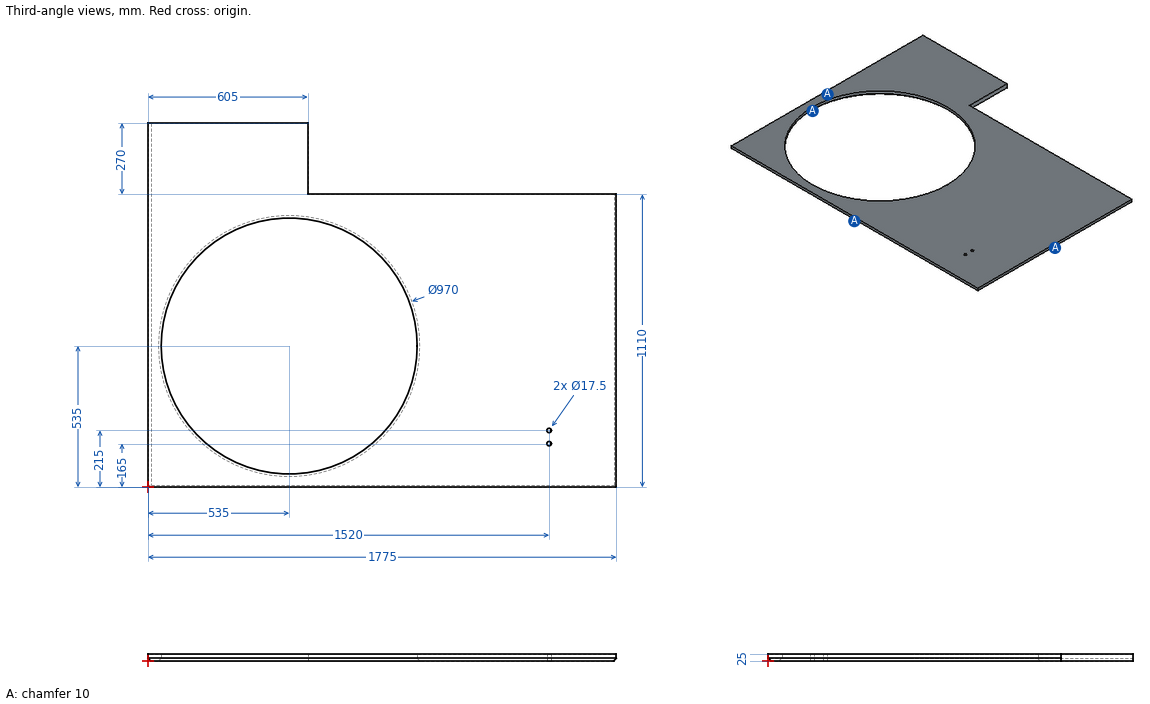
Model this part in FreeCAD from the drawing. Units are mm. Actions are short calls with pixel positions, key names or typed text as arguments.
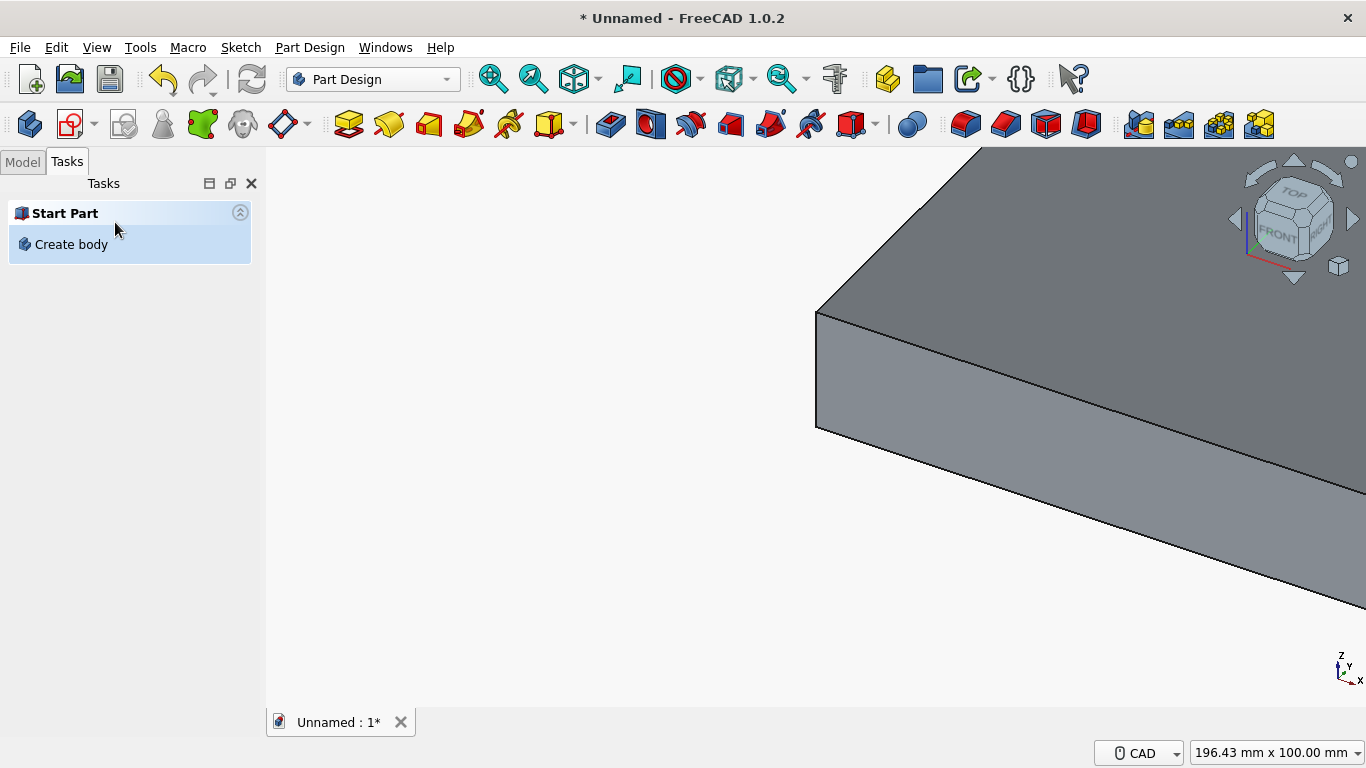
click(494, 80)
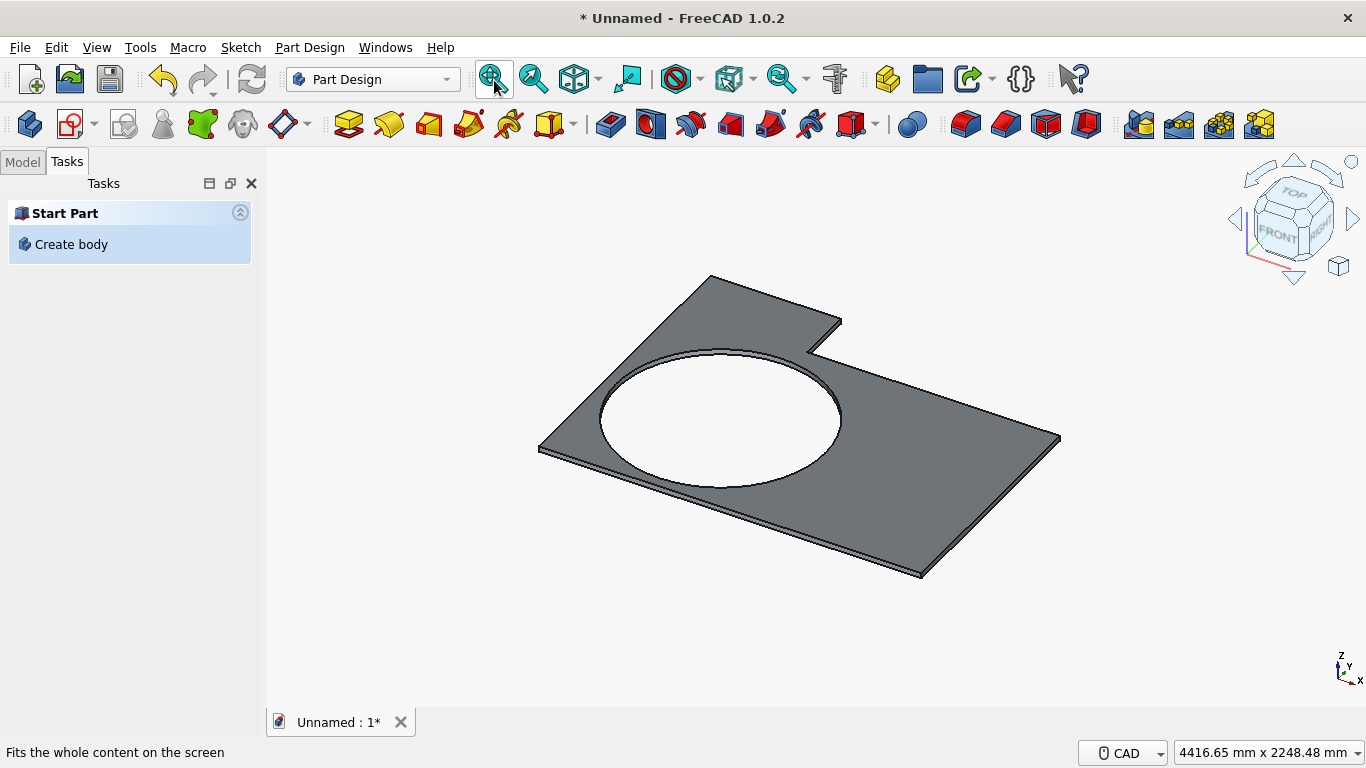
key(0)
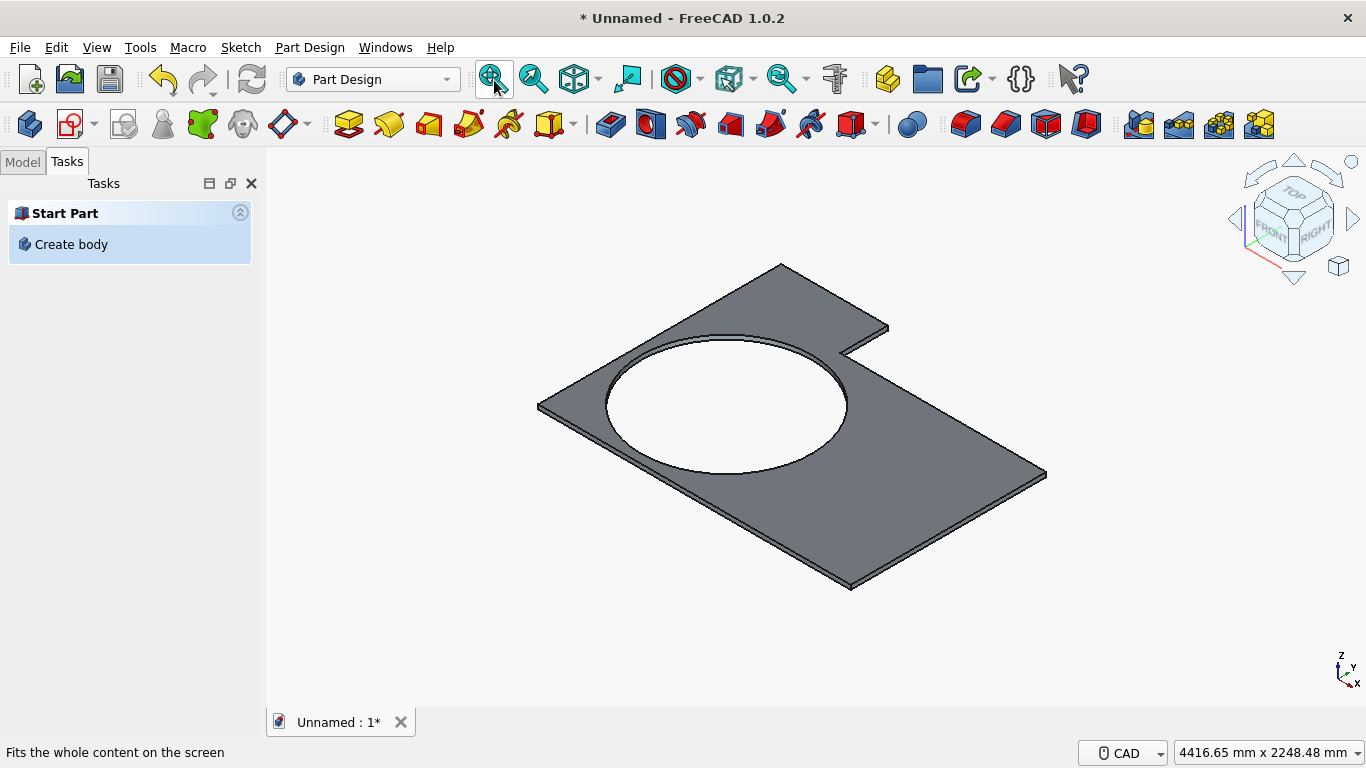
key(2)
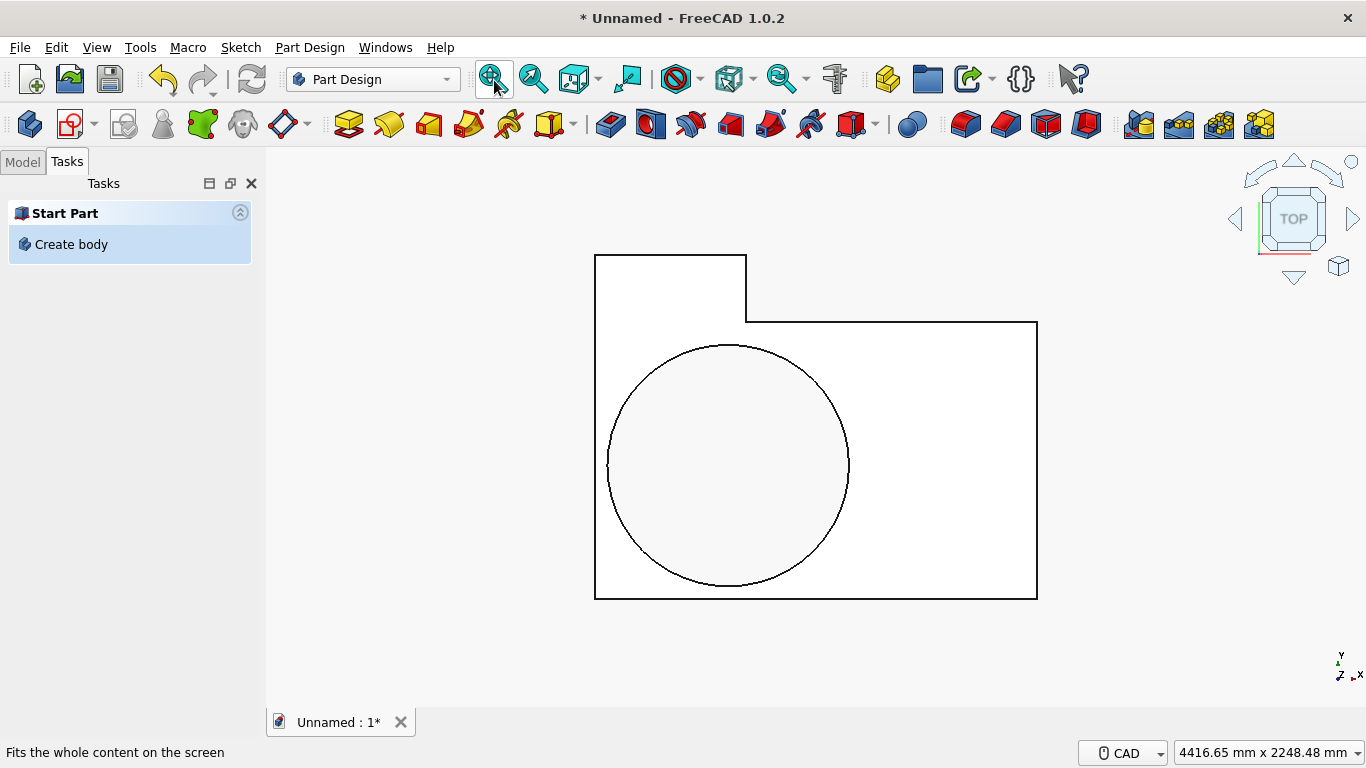
key(1)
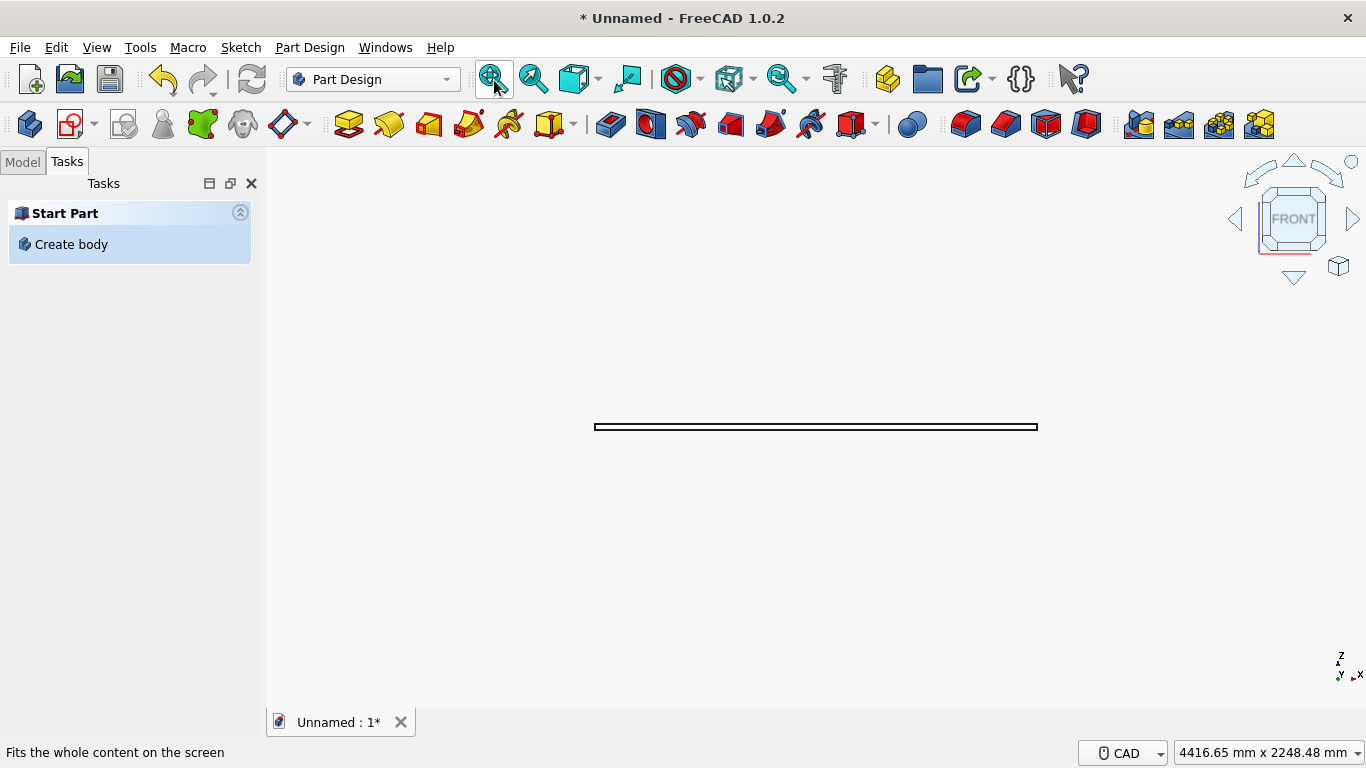
click(494, 80)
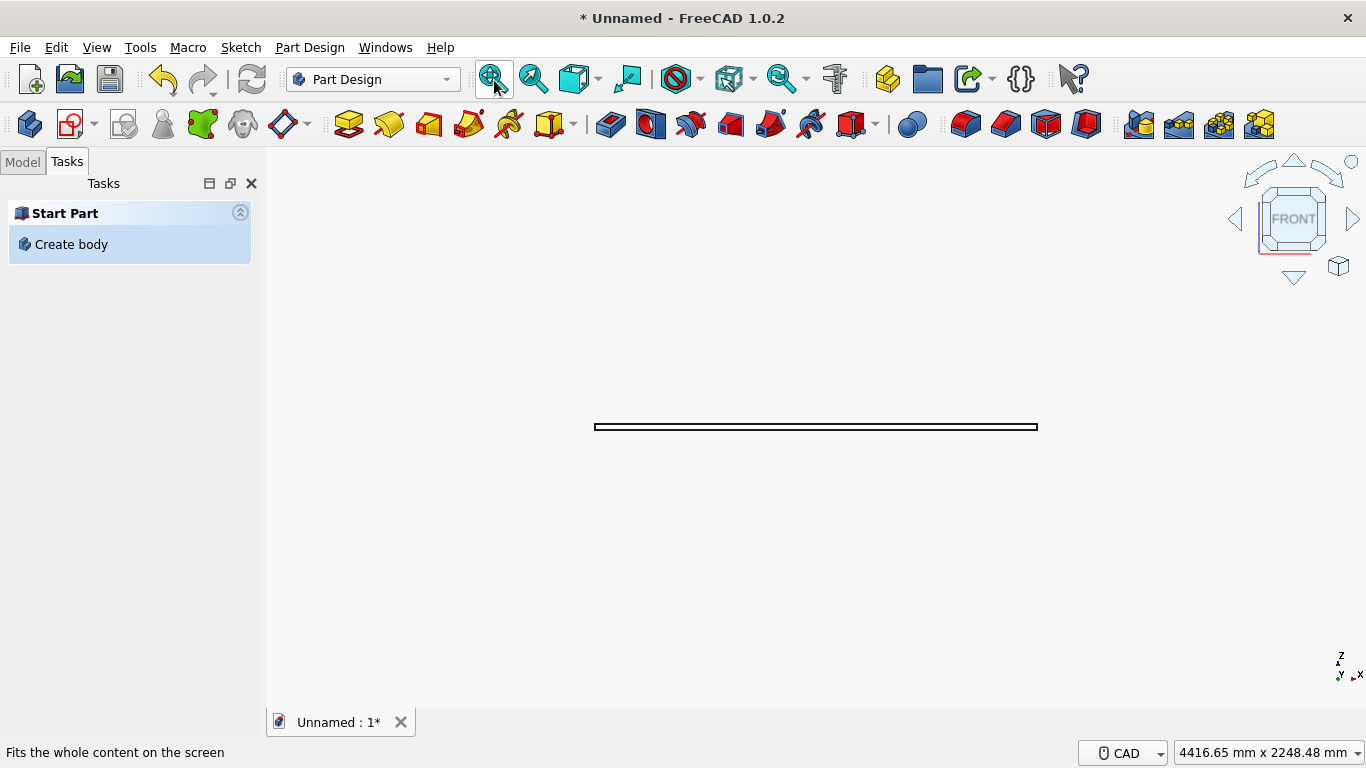
click(816, 429)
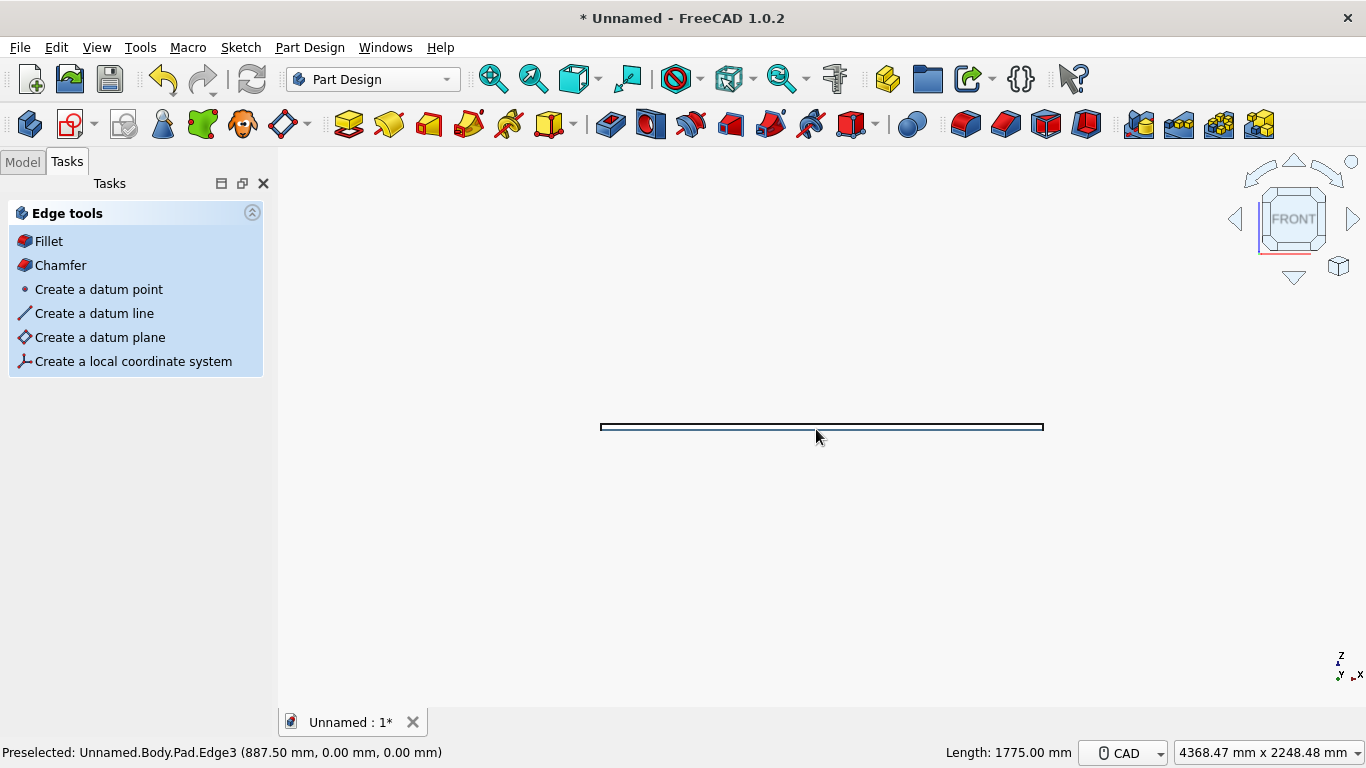
key(3)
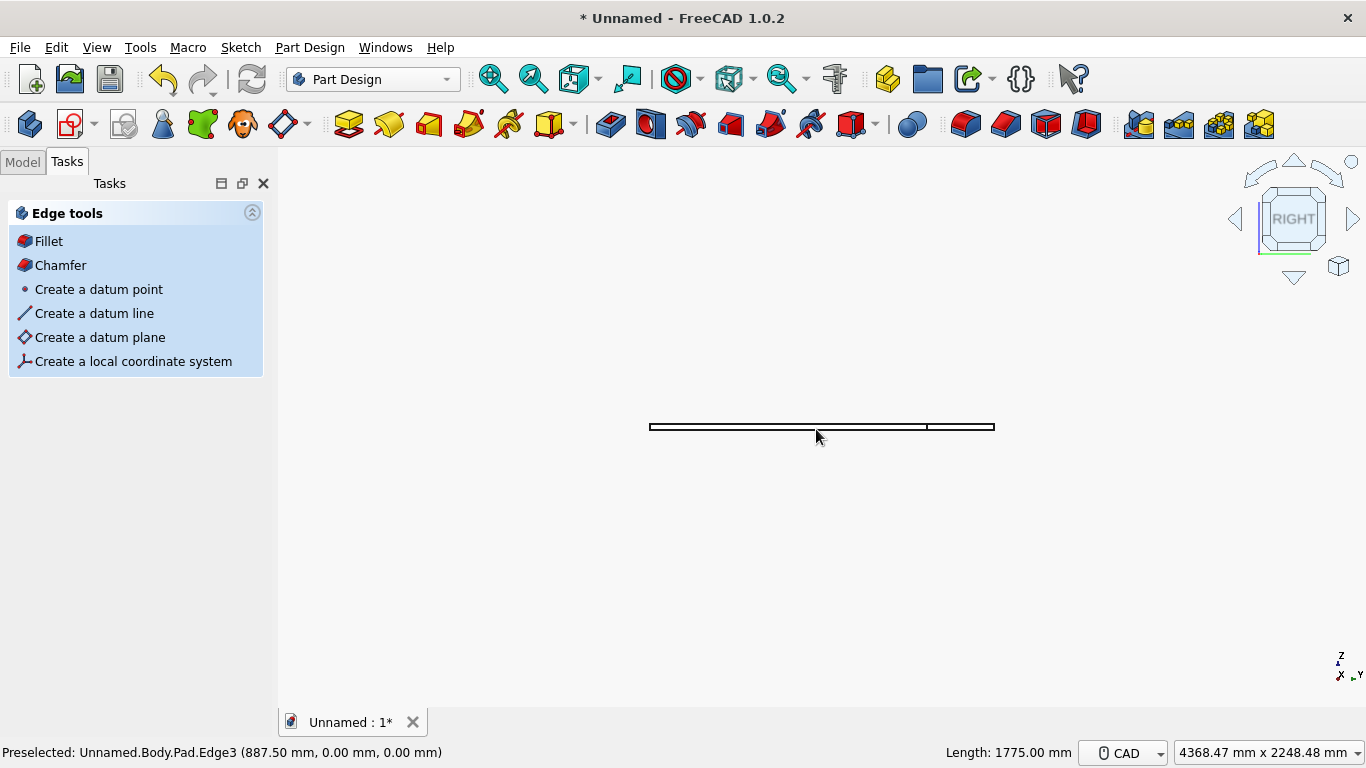
click(494, 80)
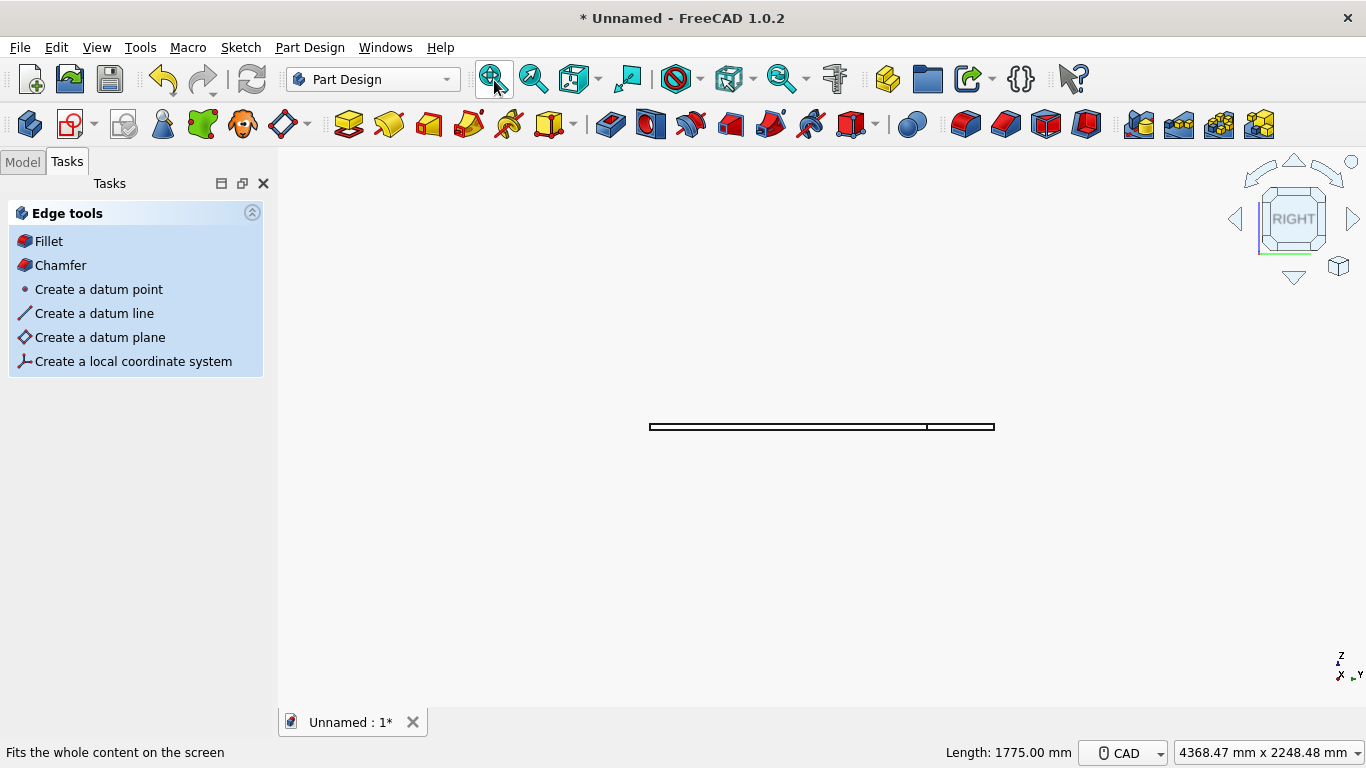
key(5)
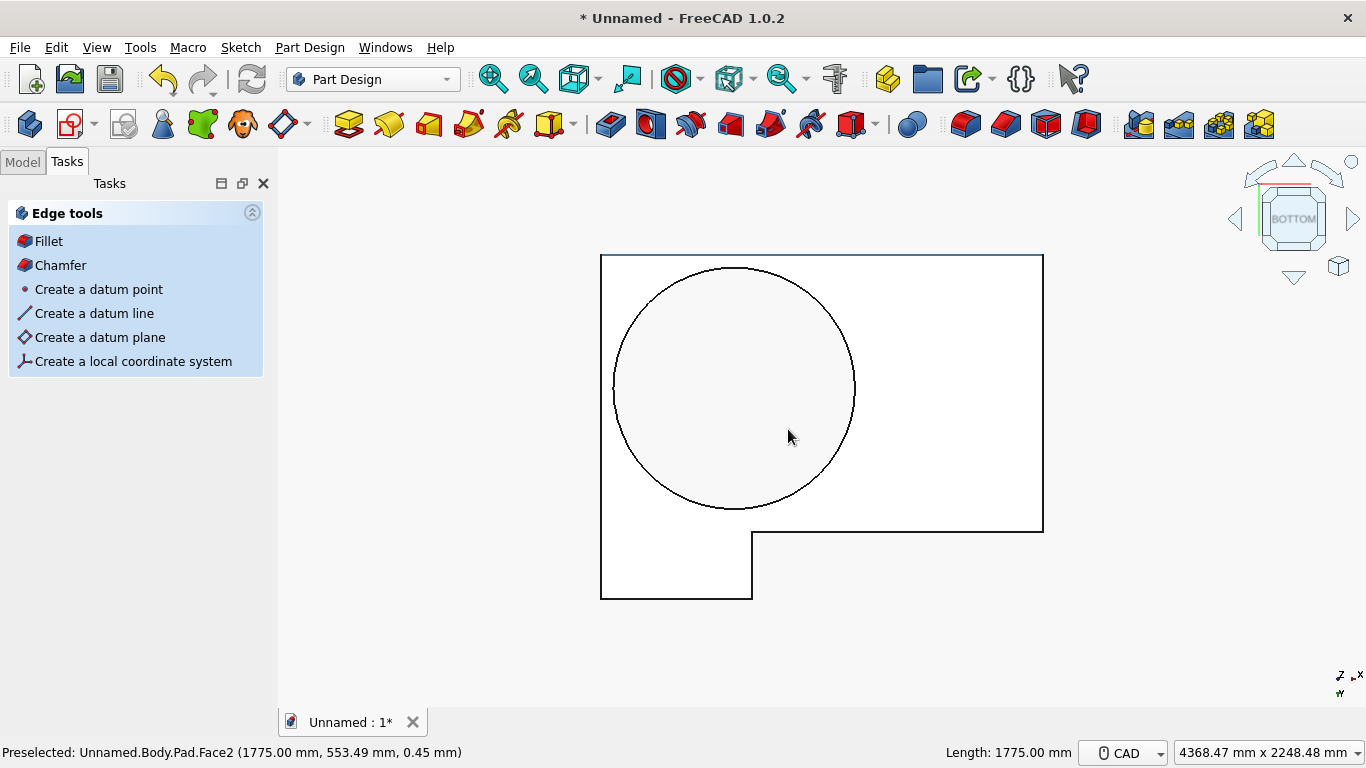
click(613, 387, ctrl)